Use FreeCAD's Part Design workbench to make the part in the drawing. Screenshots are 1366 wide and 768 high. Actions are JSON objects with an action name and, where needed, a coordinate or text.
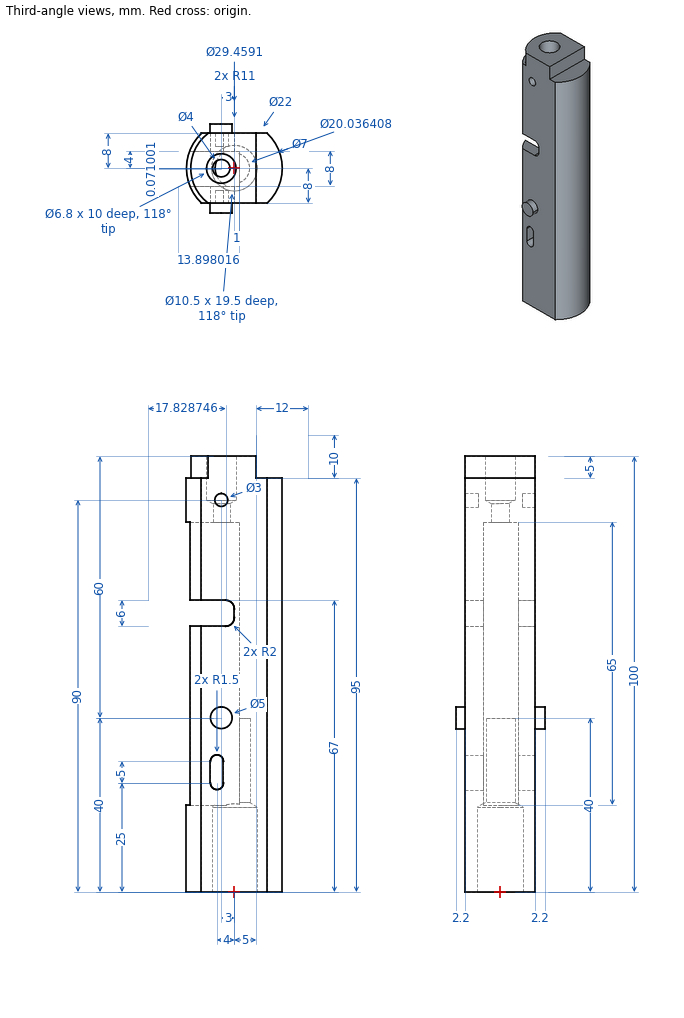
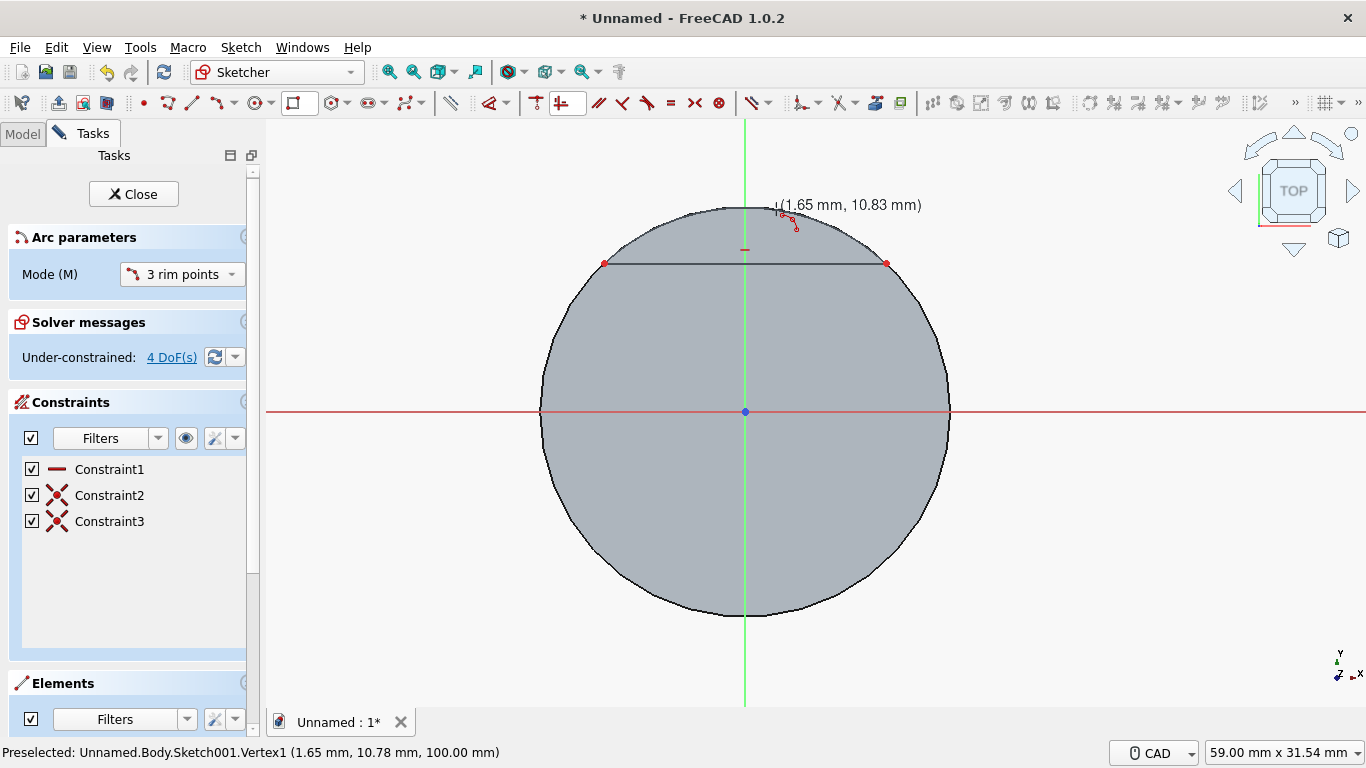
{"action": "key", "text": "g l"}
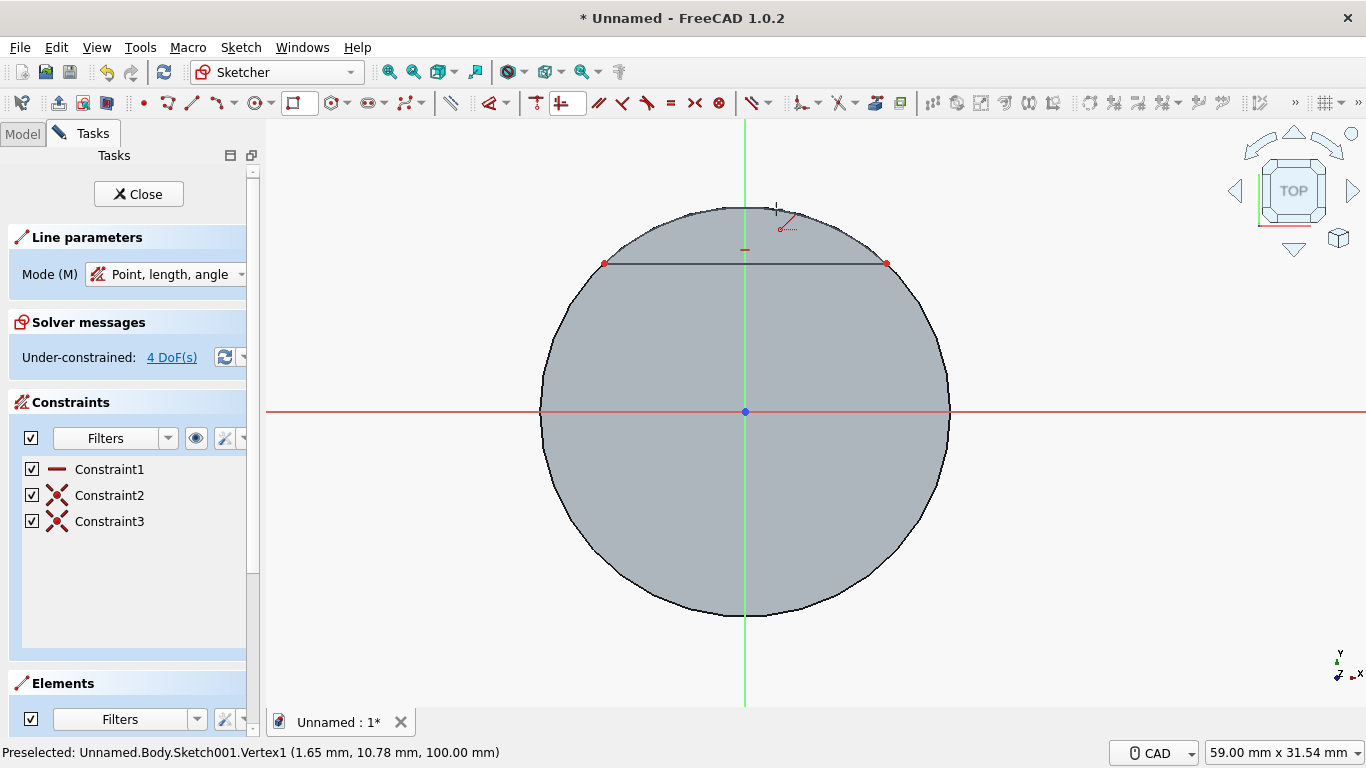
{"action": "left_click", "coordinate": [886, 561]}
{"action": "left_click", "coordinate": [604, 561]}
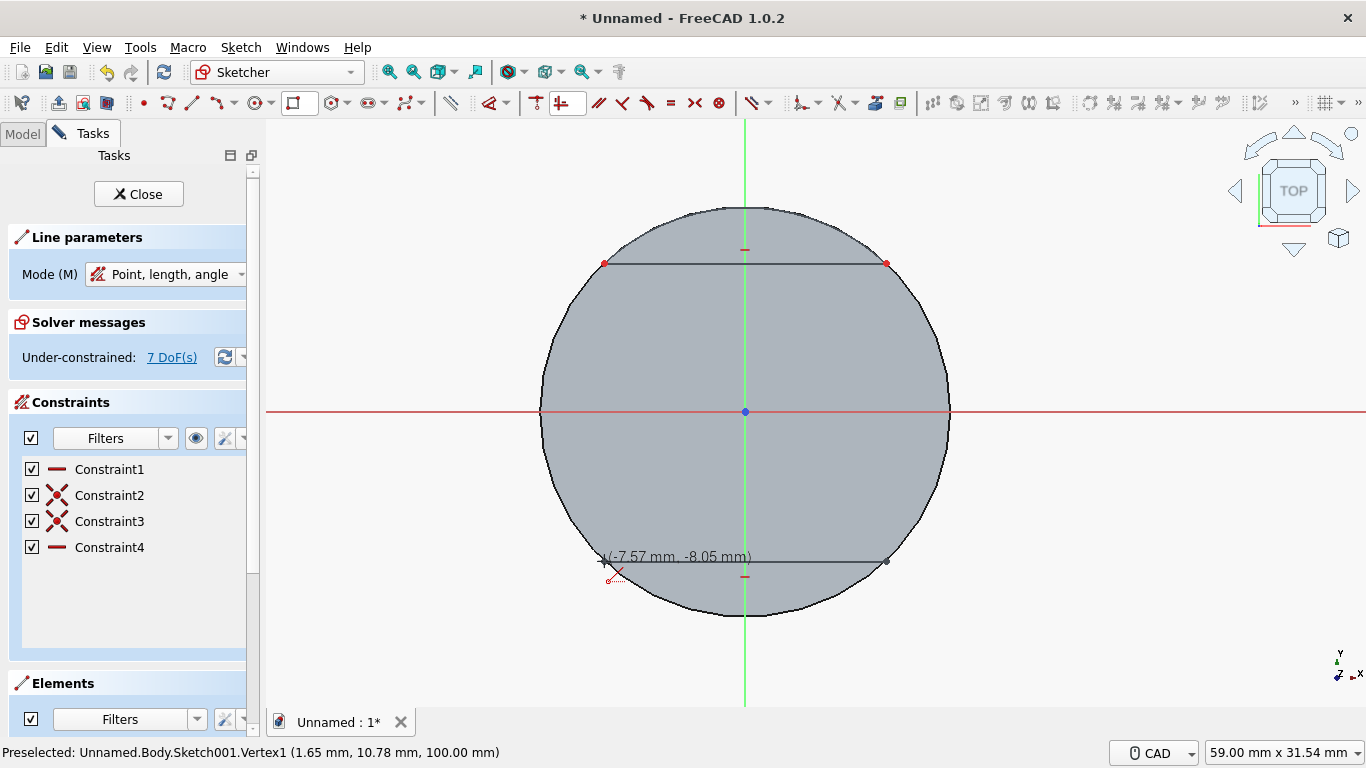
{"action": "key", "text": "g 3 a"}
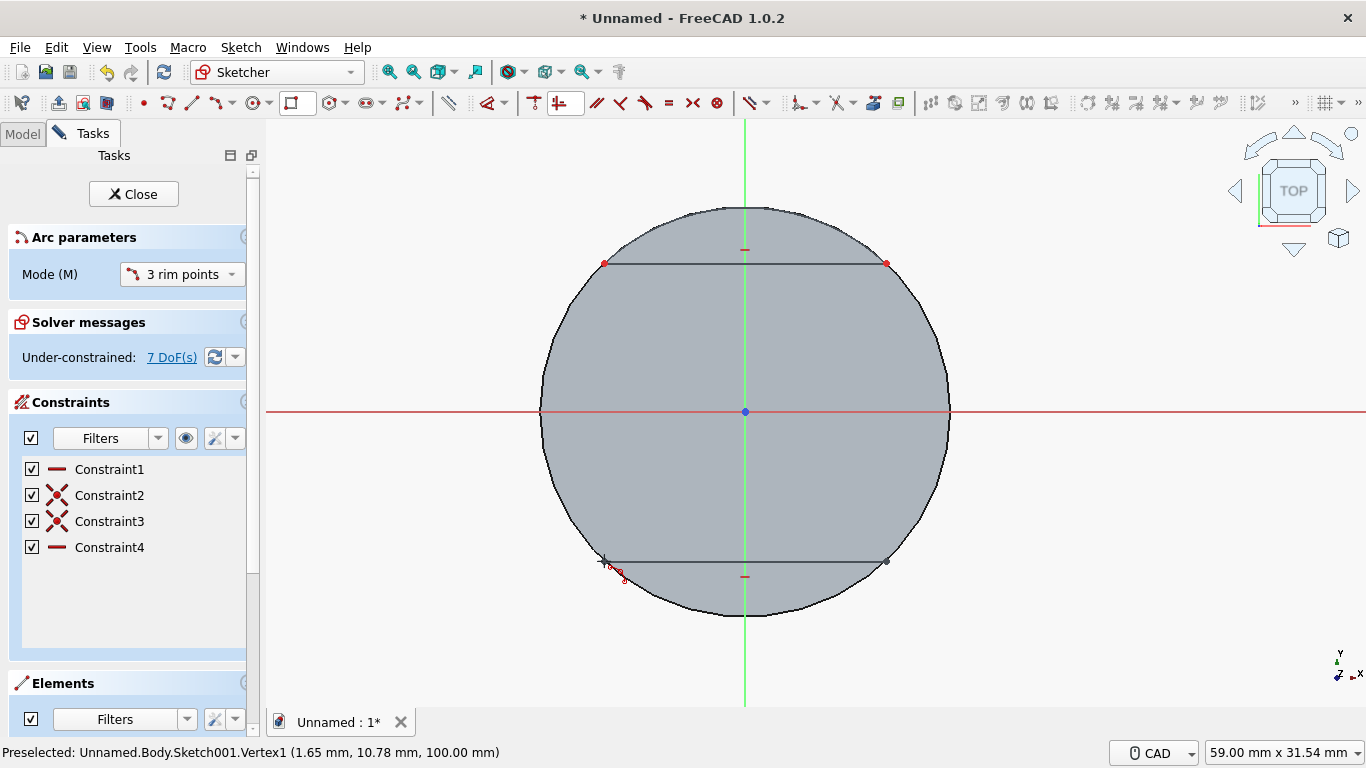
{"action": "left_click", "coordinate": [604, 562]}
{"action": "left_click", "coordinate": [886, 562]}
{"action": "left_click", "coordinate": [714, 615]}
{"action": "key", "text": "Escape"}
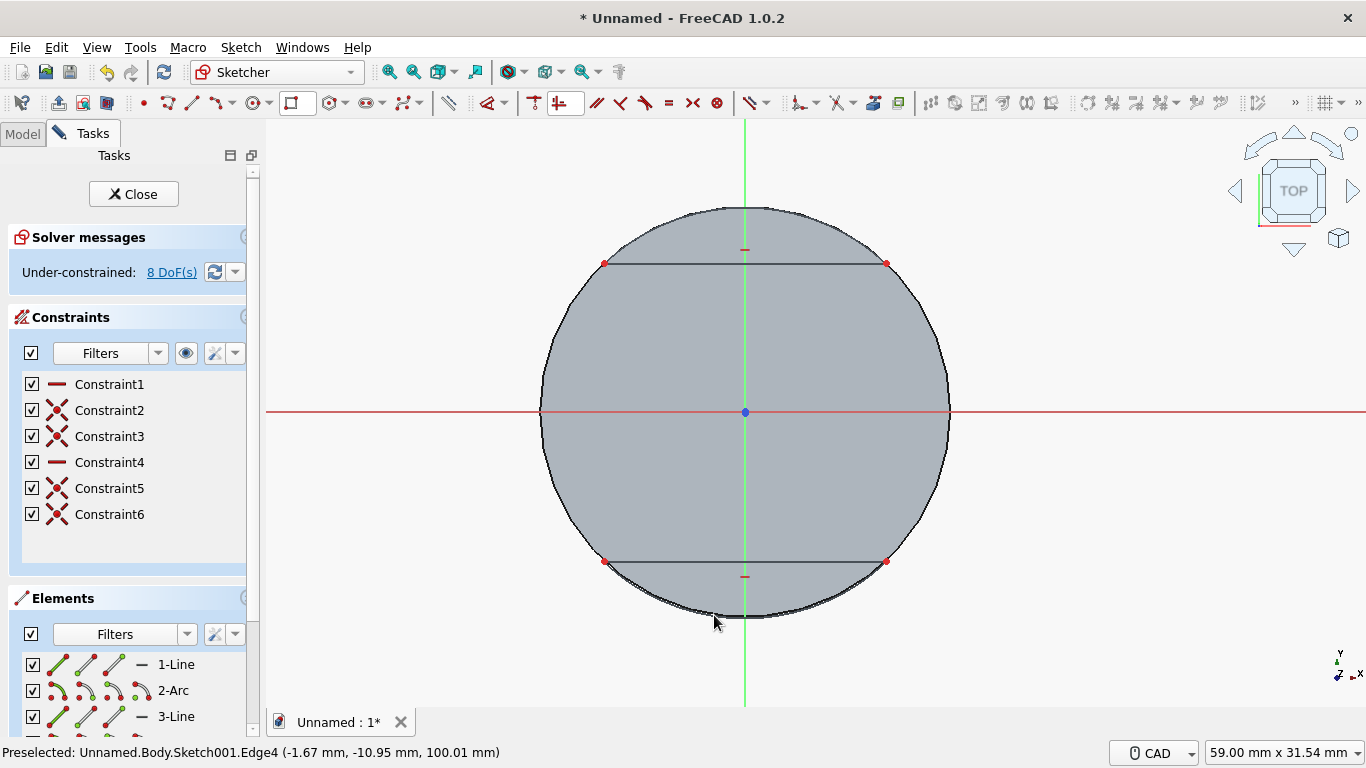
{"action": "left_click", "coordinate": [806, 217]}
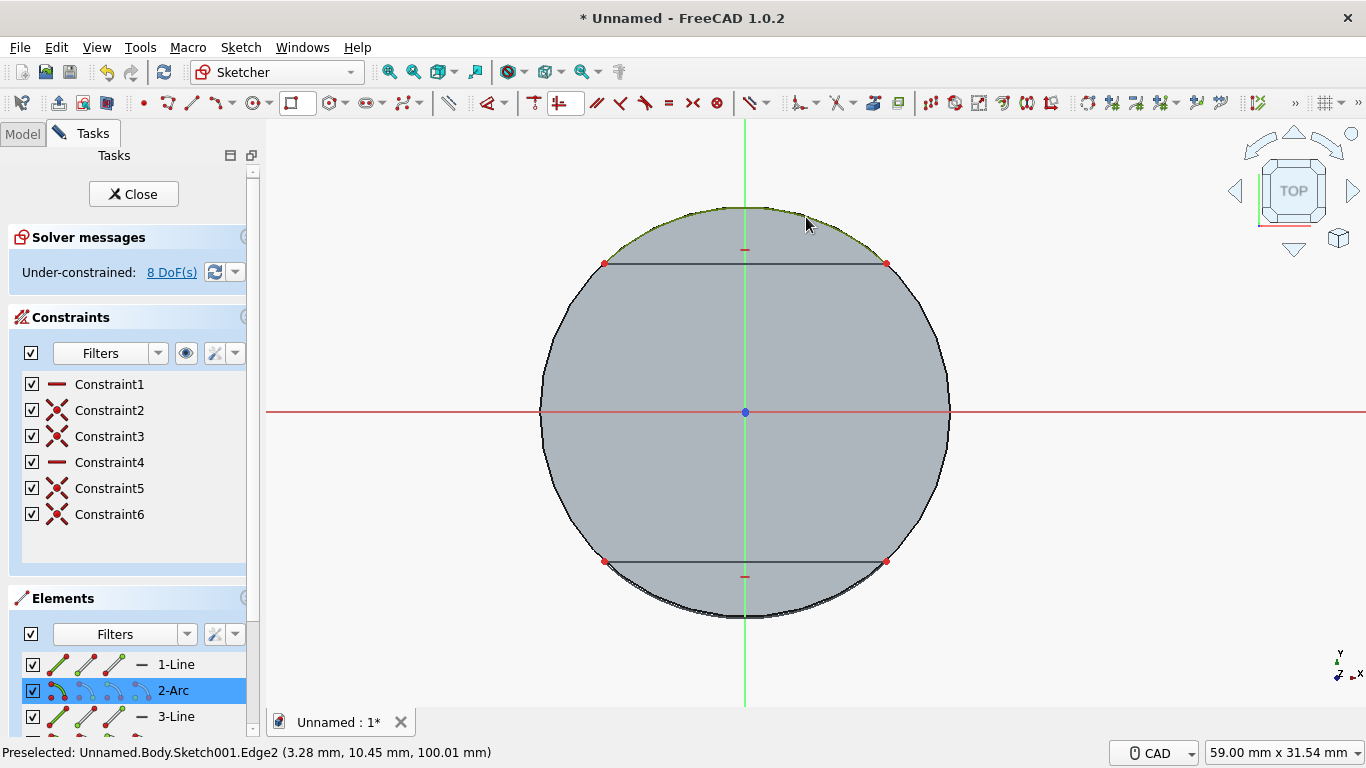
{"action": "left_click", "coordinate": [684, 609]}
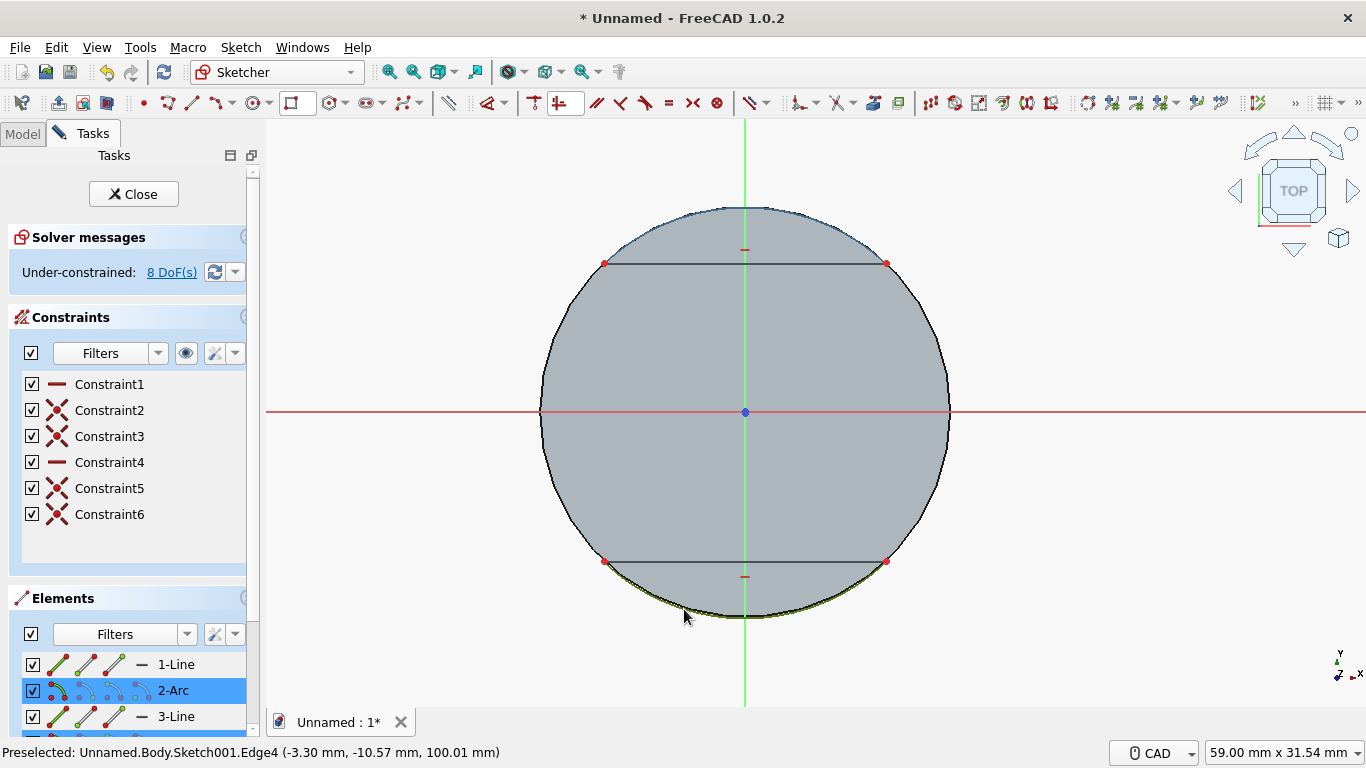
{"action": "left_click", "coordinate": [534, 104]}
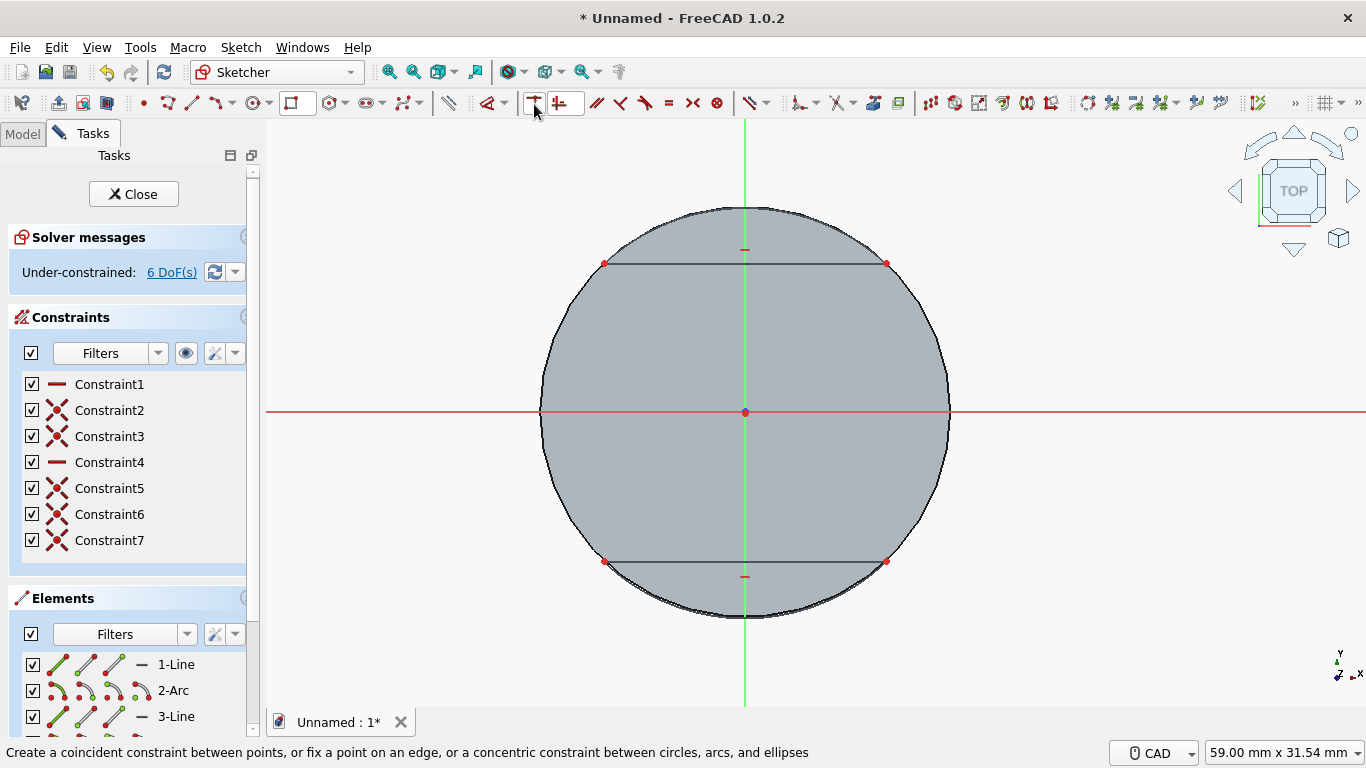
{"action": "left_click_drag", "start_coordinate": [735, 402], "coordinate": [755, 424]}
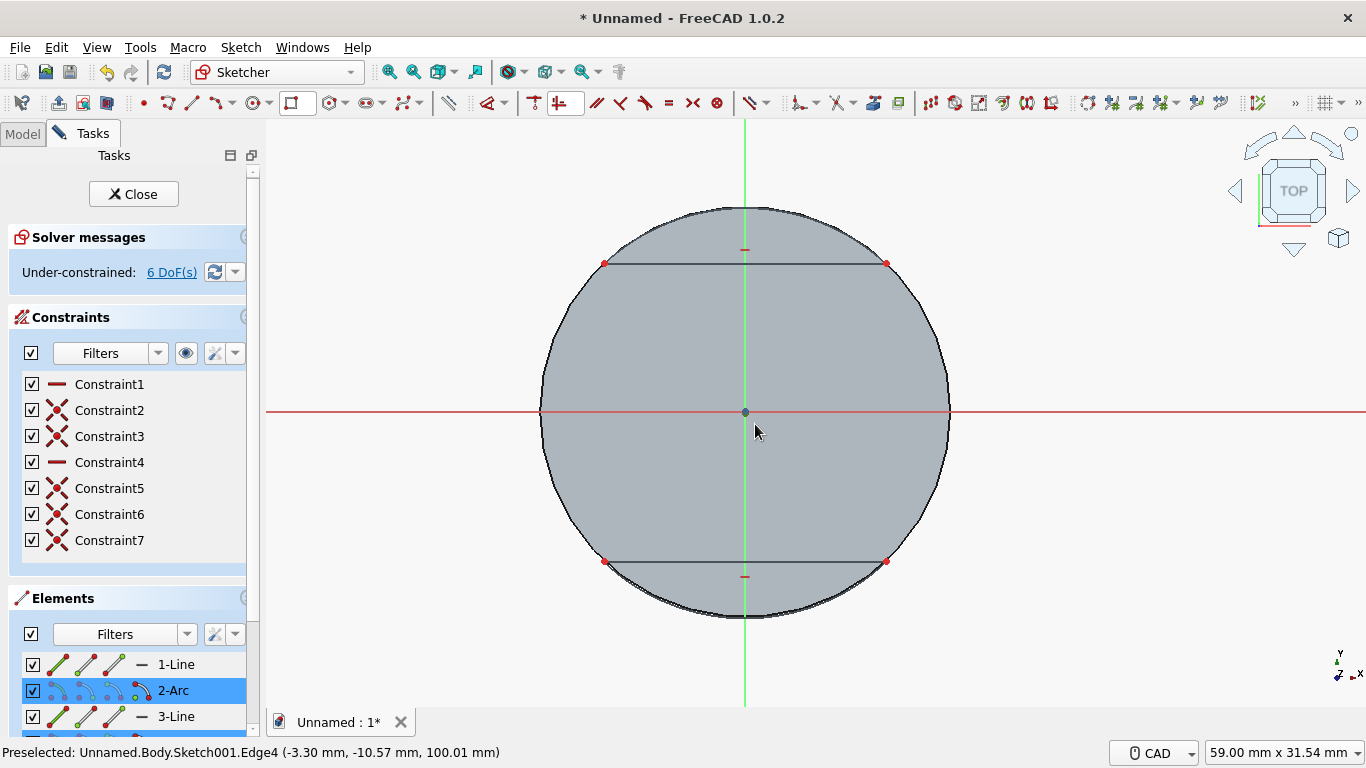
{"action": "key", "text": "c"}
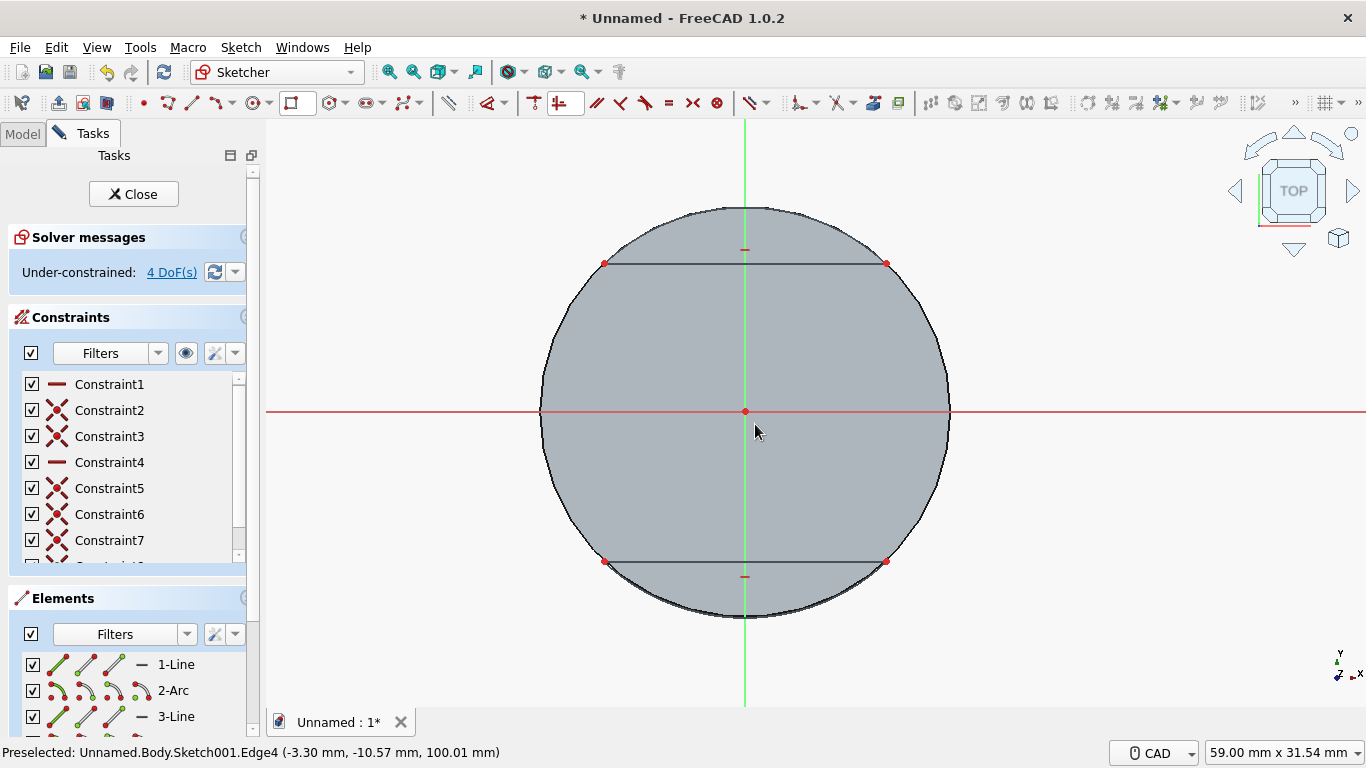
{"action": "left_click", "coordinate": [806, 217]}